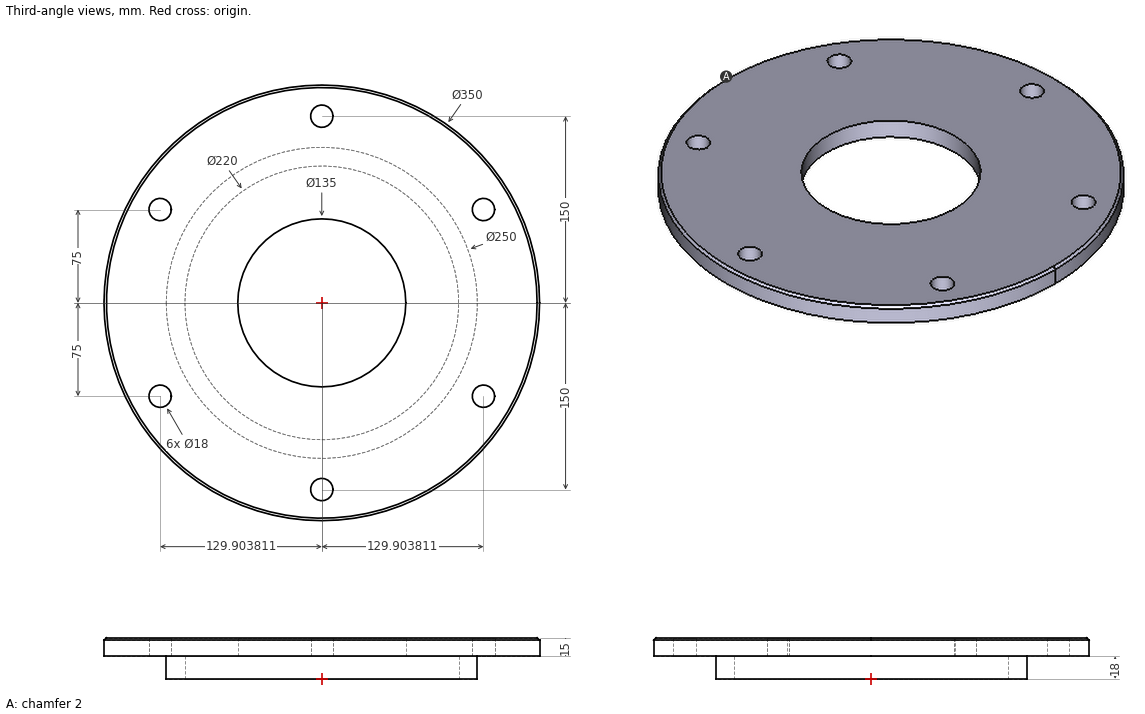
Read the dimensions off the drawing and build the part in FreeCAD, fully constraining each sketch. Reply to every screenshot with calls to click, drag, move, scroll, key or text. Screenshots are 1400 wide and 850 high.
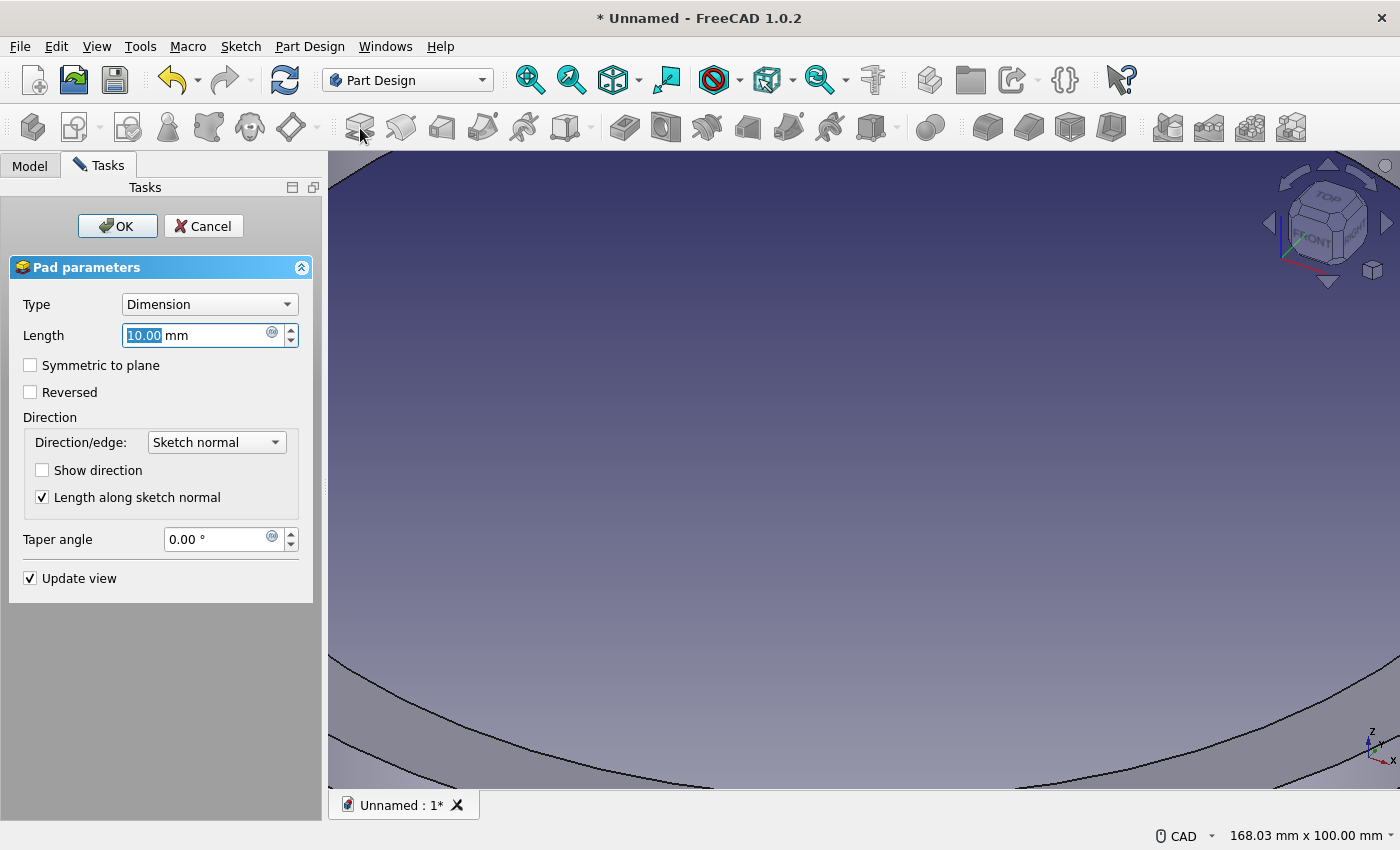
text(18)
key(Tab)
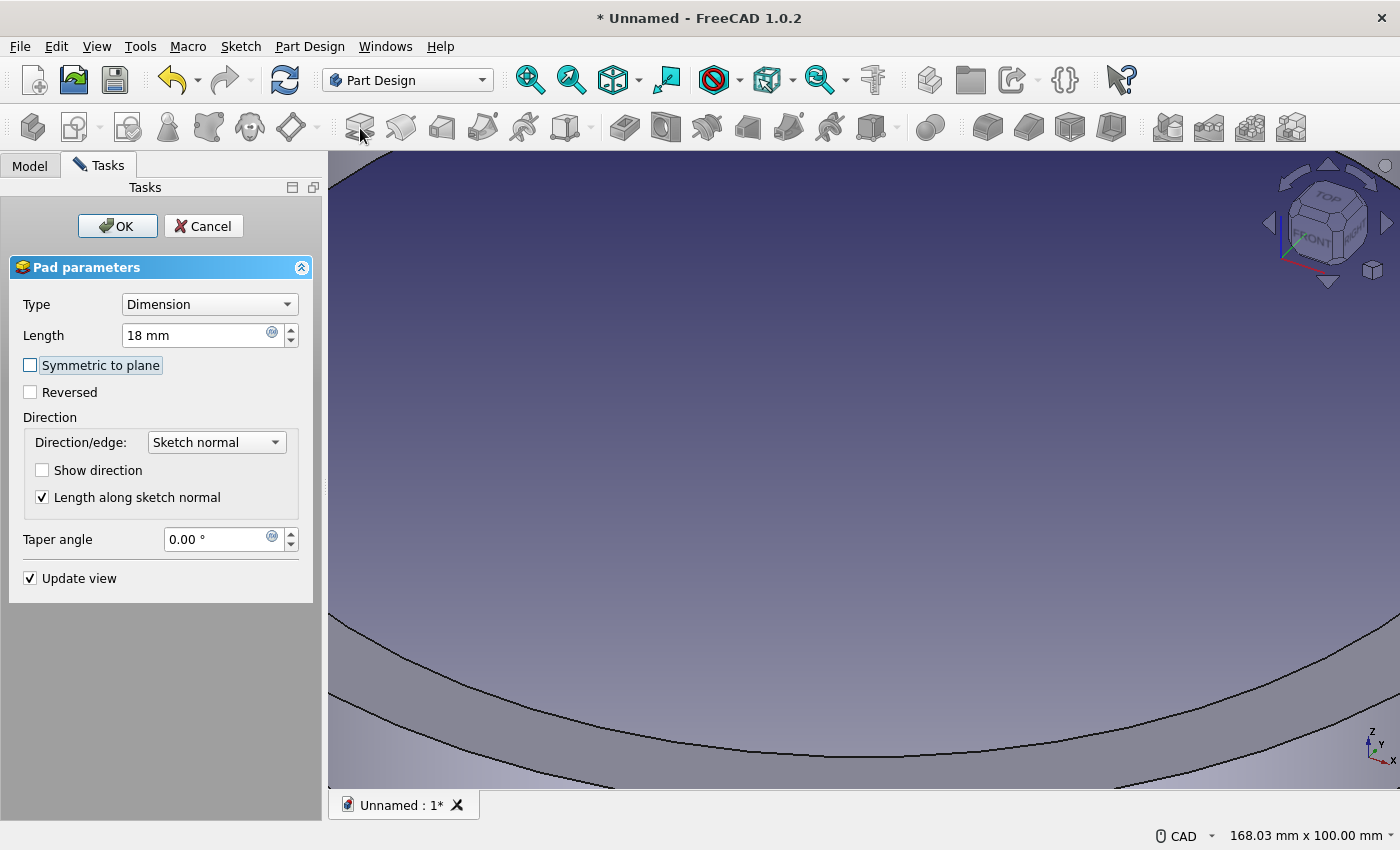
click(118, 226)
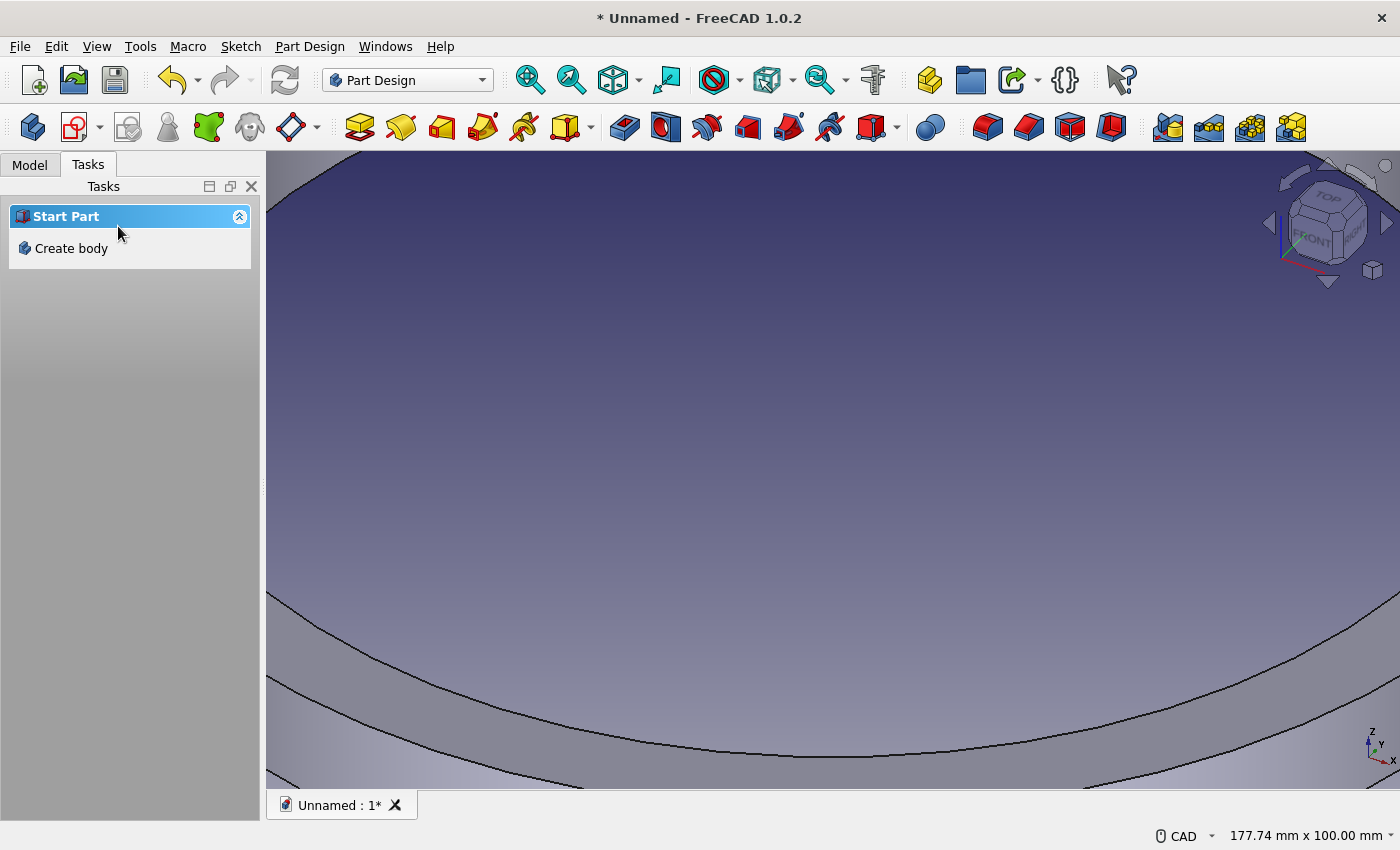
click(531, 80)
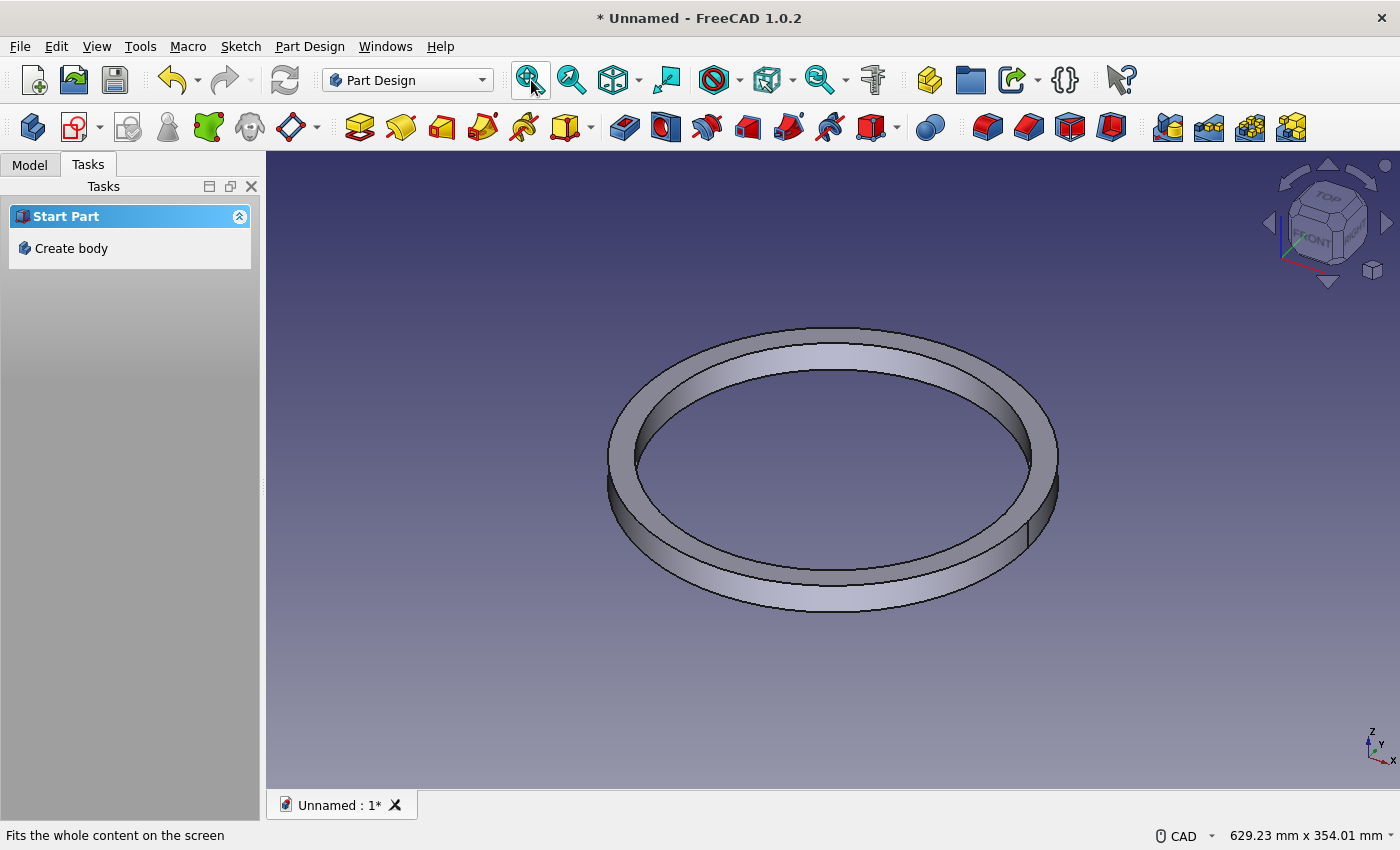
scroll(698, 368, up, 5)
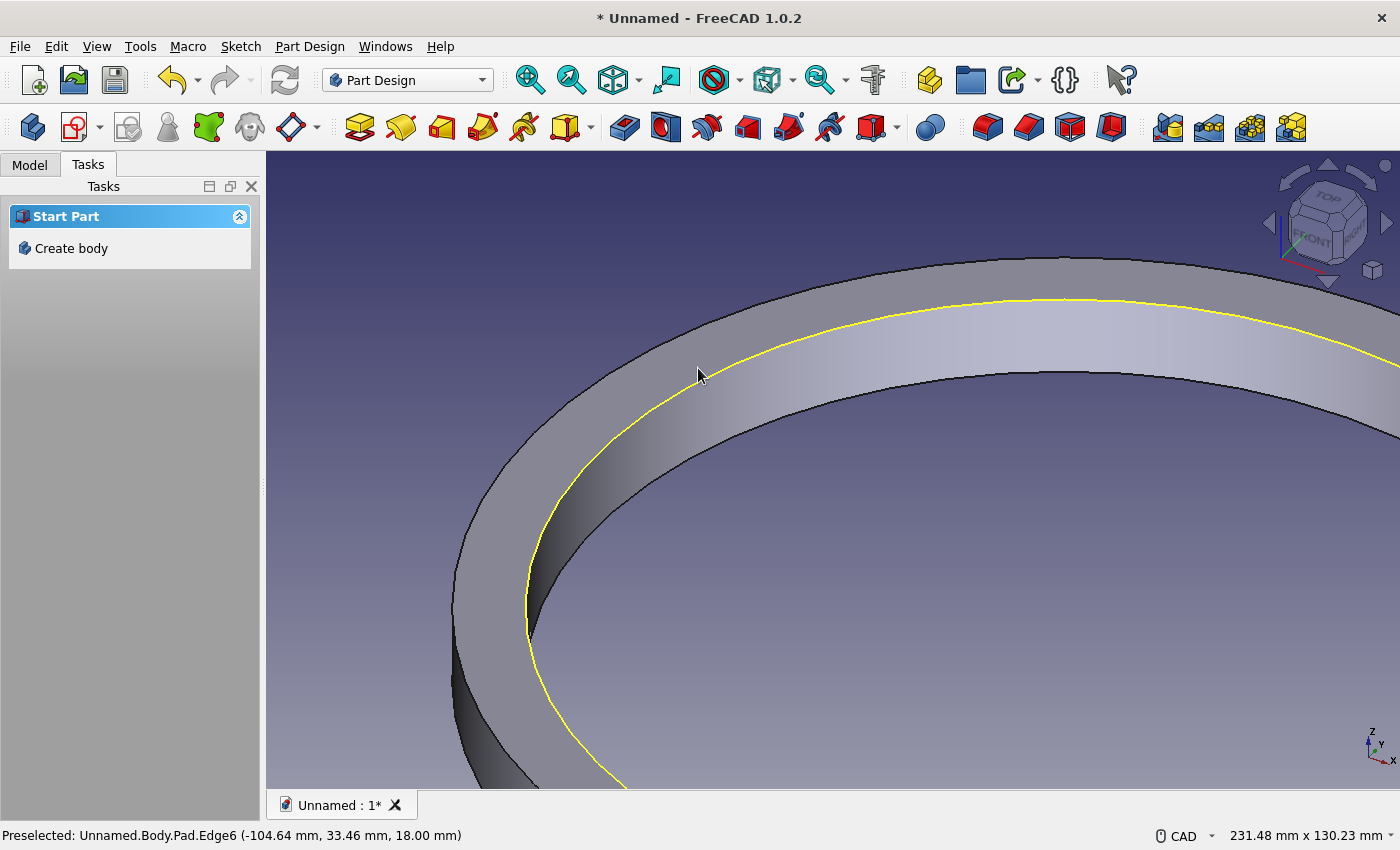
click(697, 370)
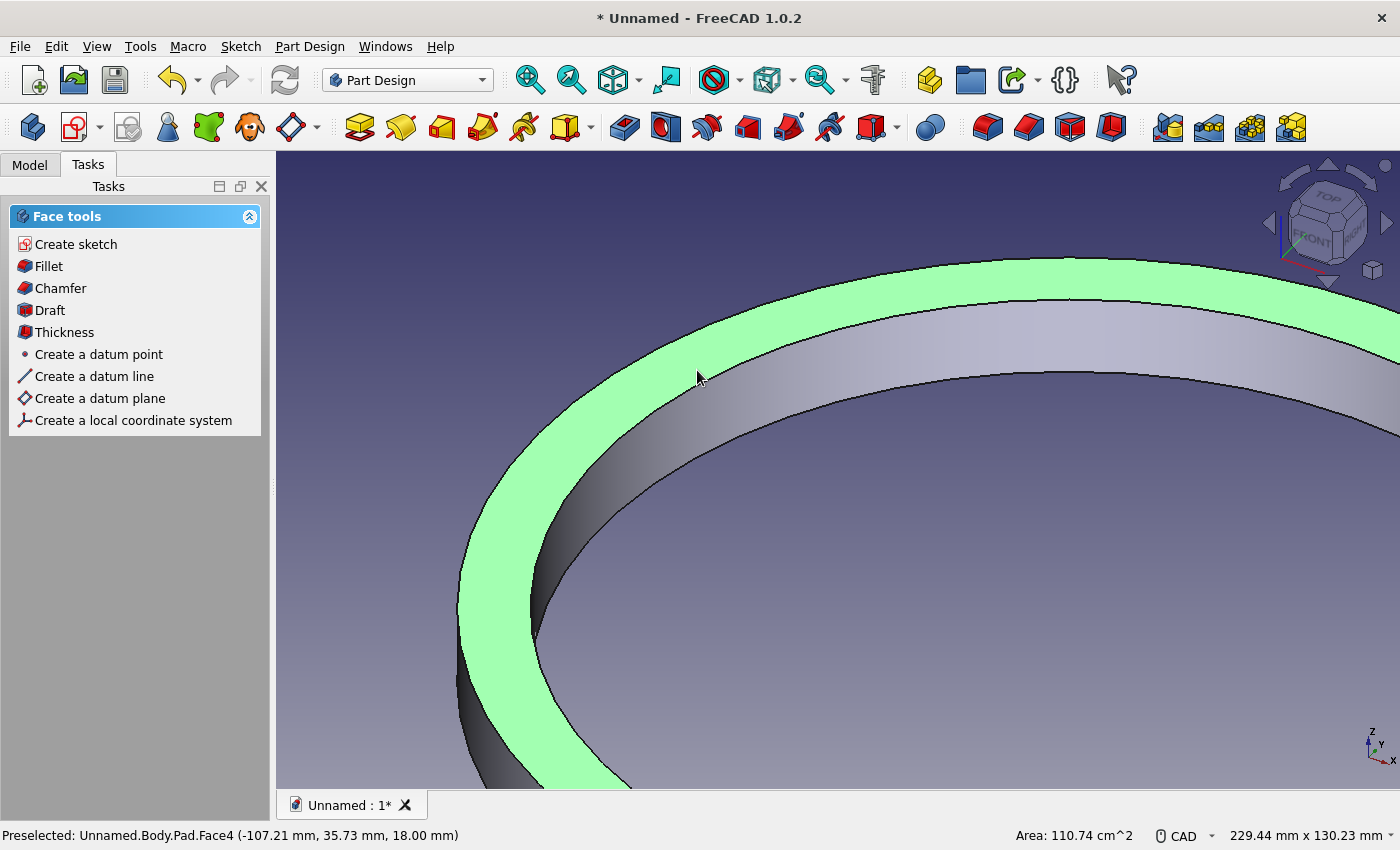
click(74, 128)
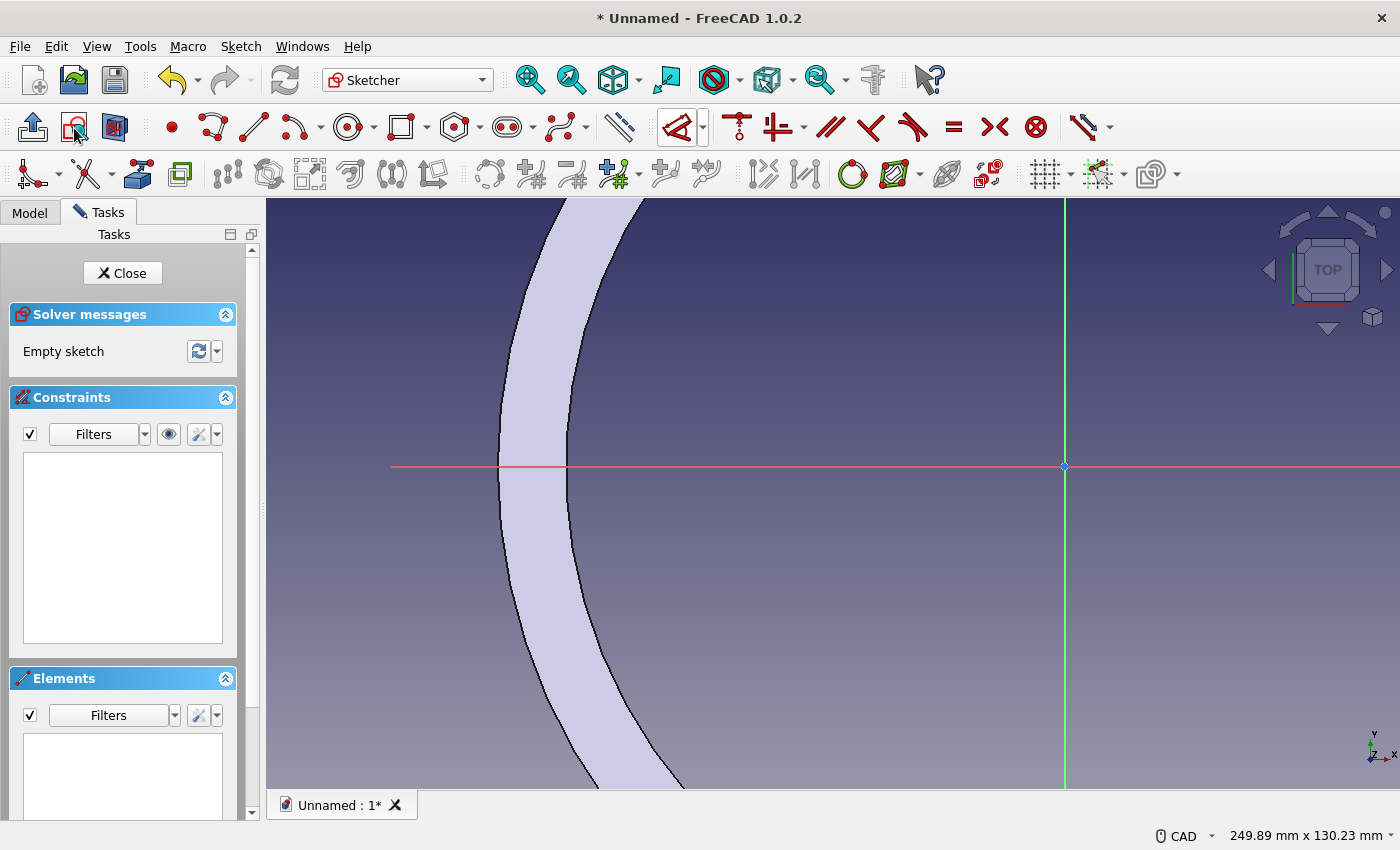
scroll(666, 502, down, 7)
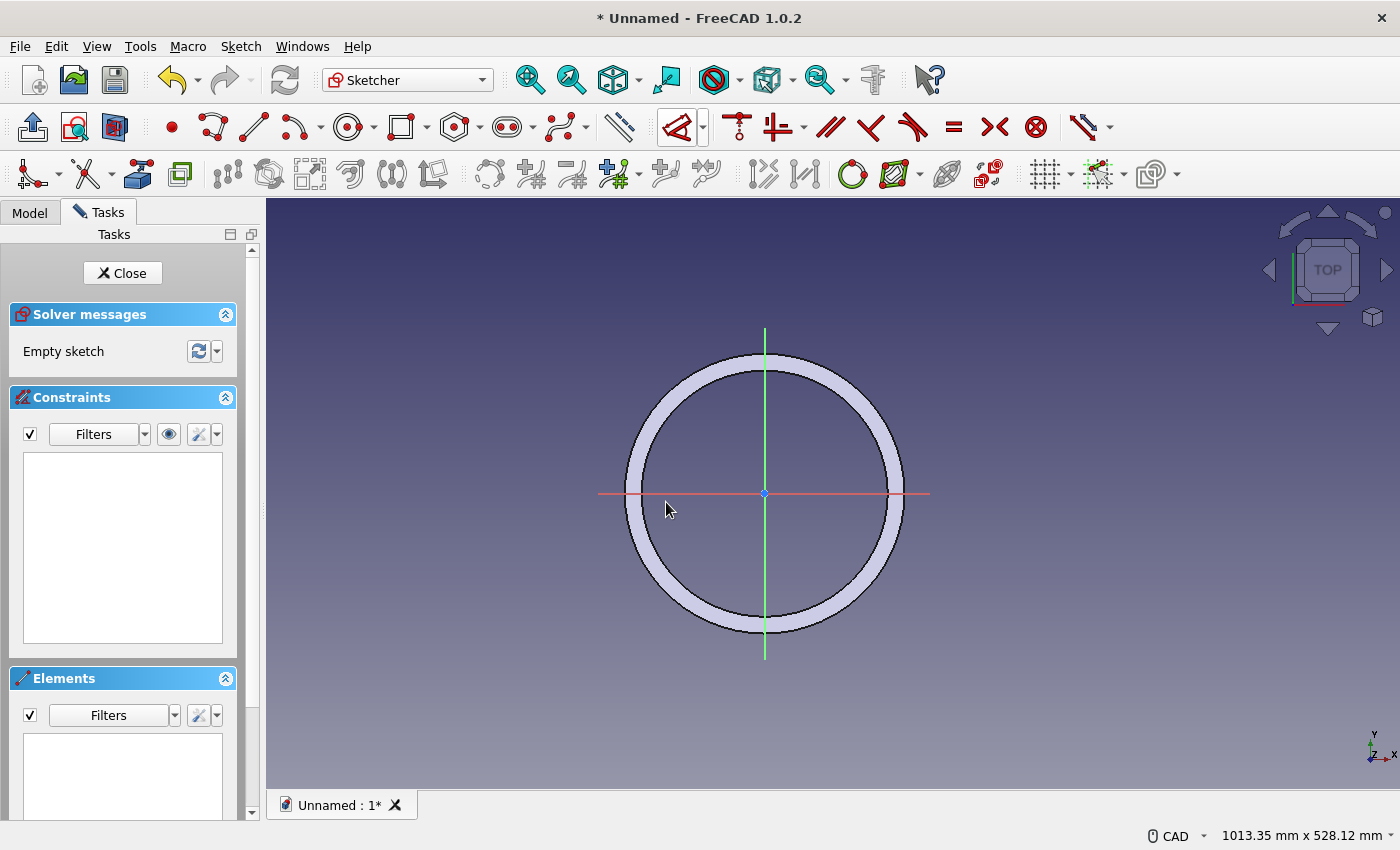
key(g)
key(c)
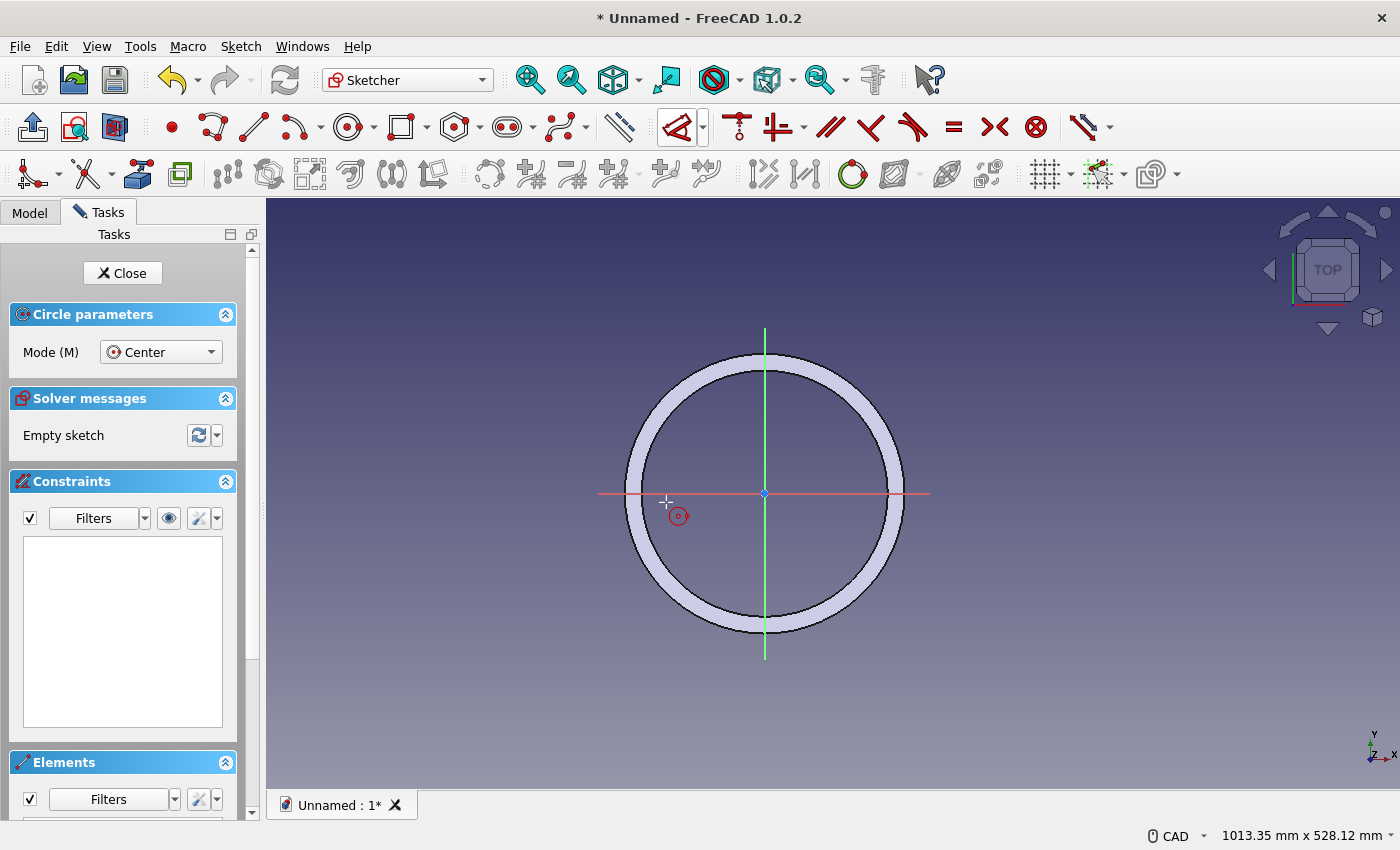
click(765, 494)
click(903, 355)